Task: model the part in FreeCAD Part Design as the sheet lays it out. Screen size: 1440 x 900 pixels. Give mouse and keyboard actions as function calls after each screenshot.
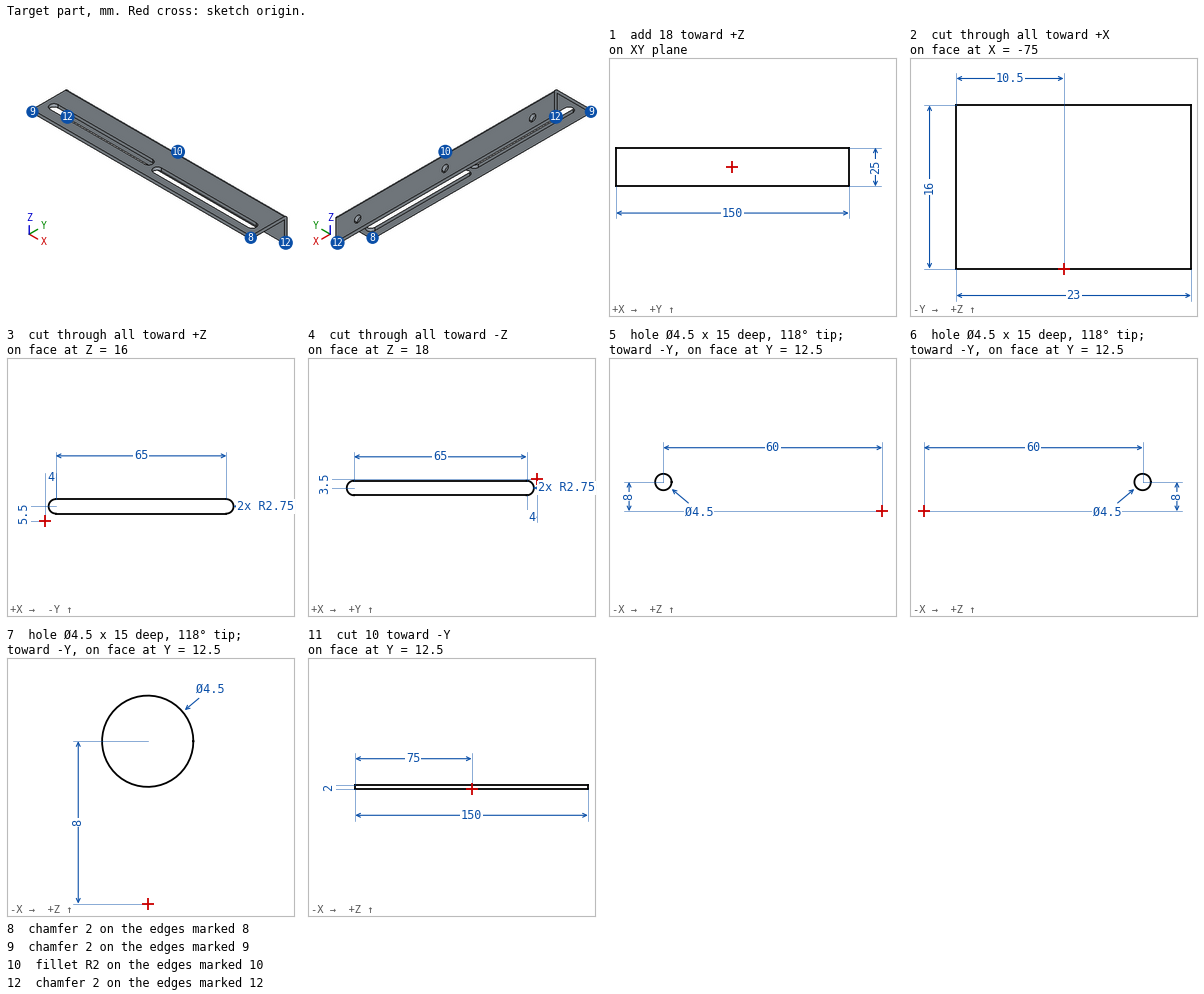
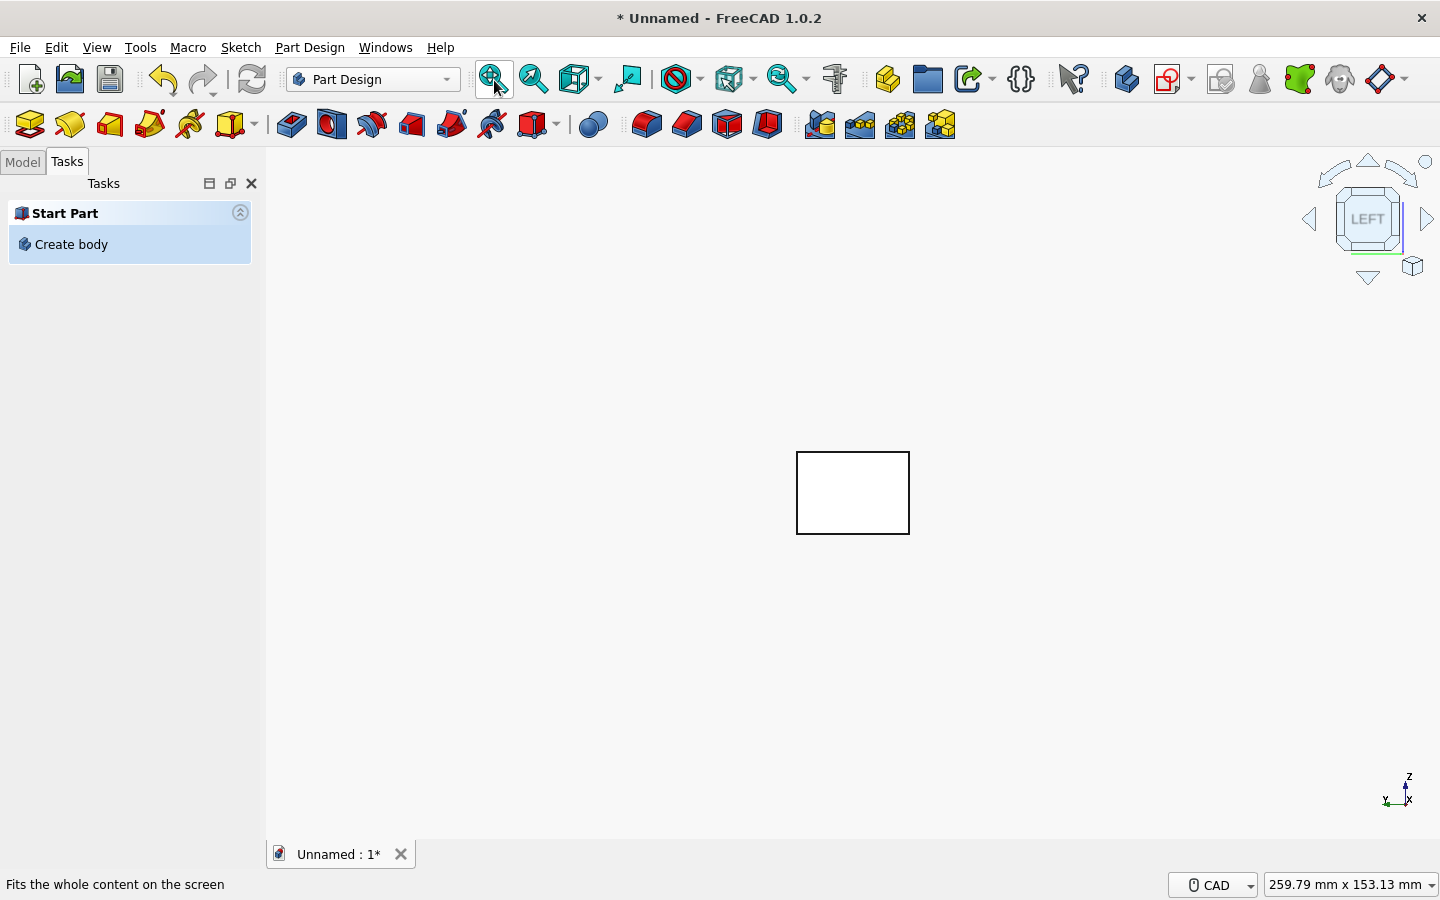
click(853, 492)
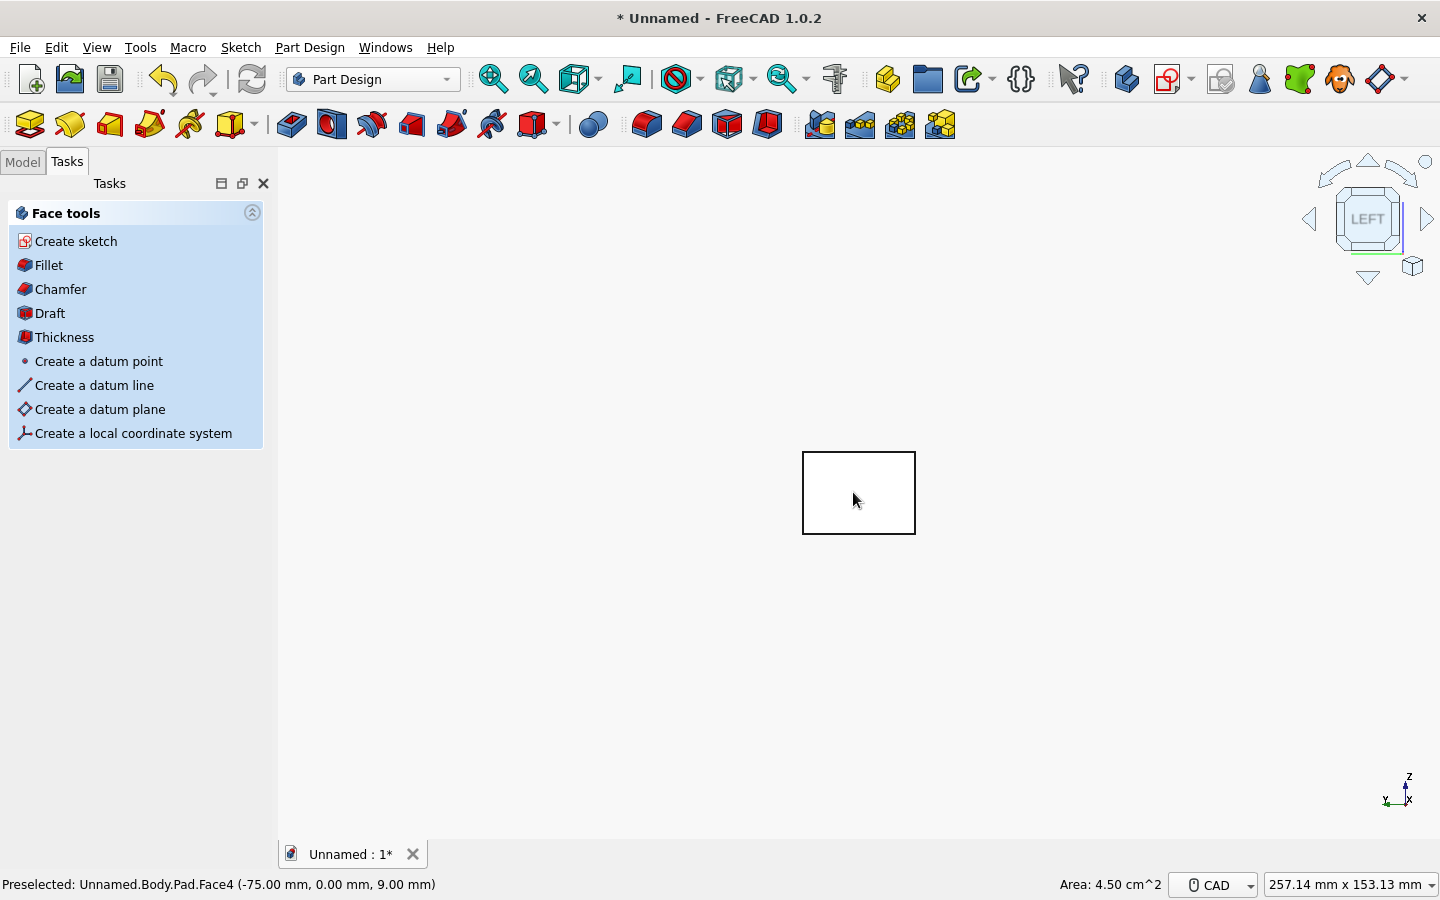
click(1168, 80)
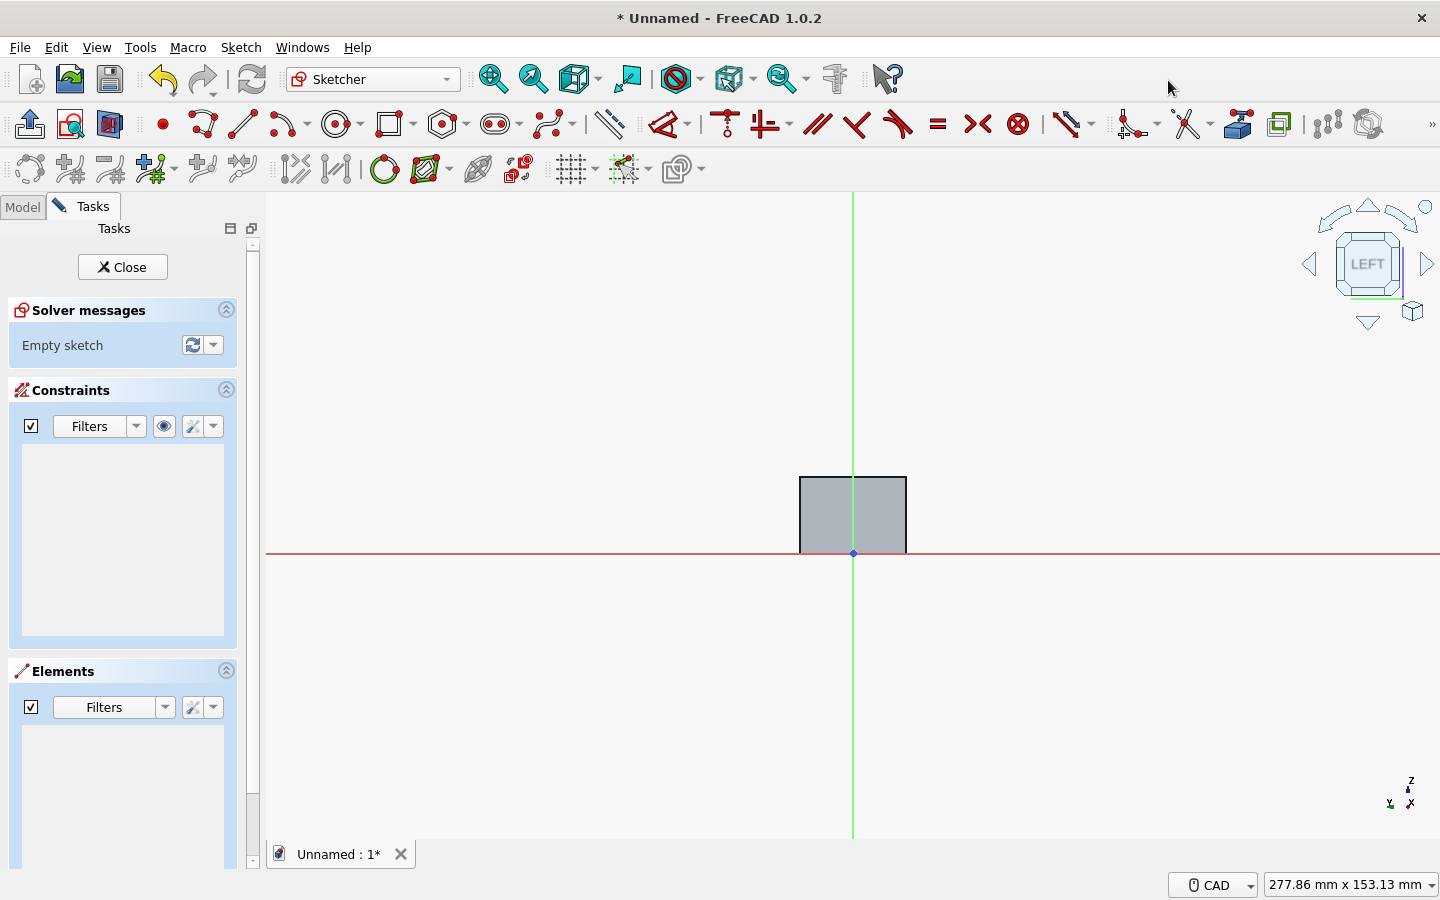
scroll(872, 521, up, 9)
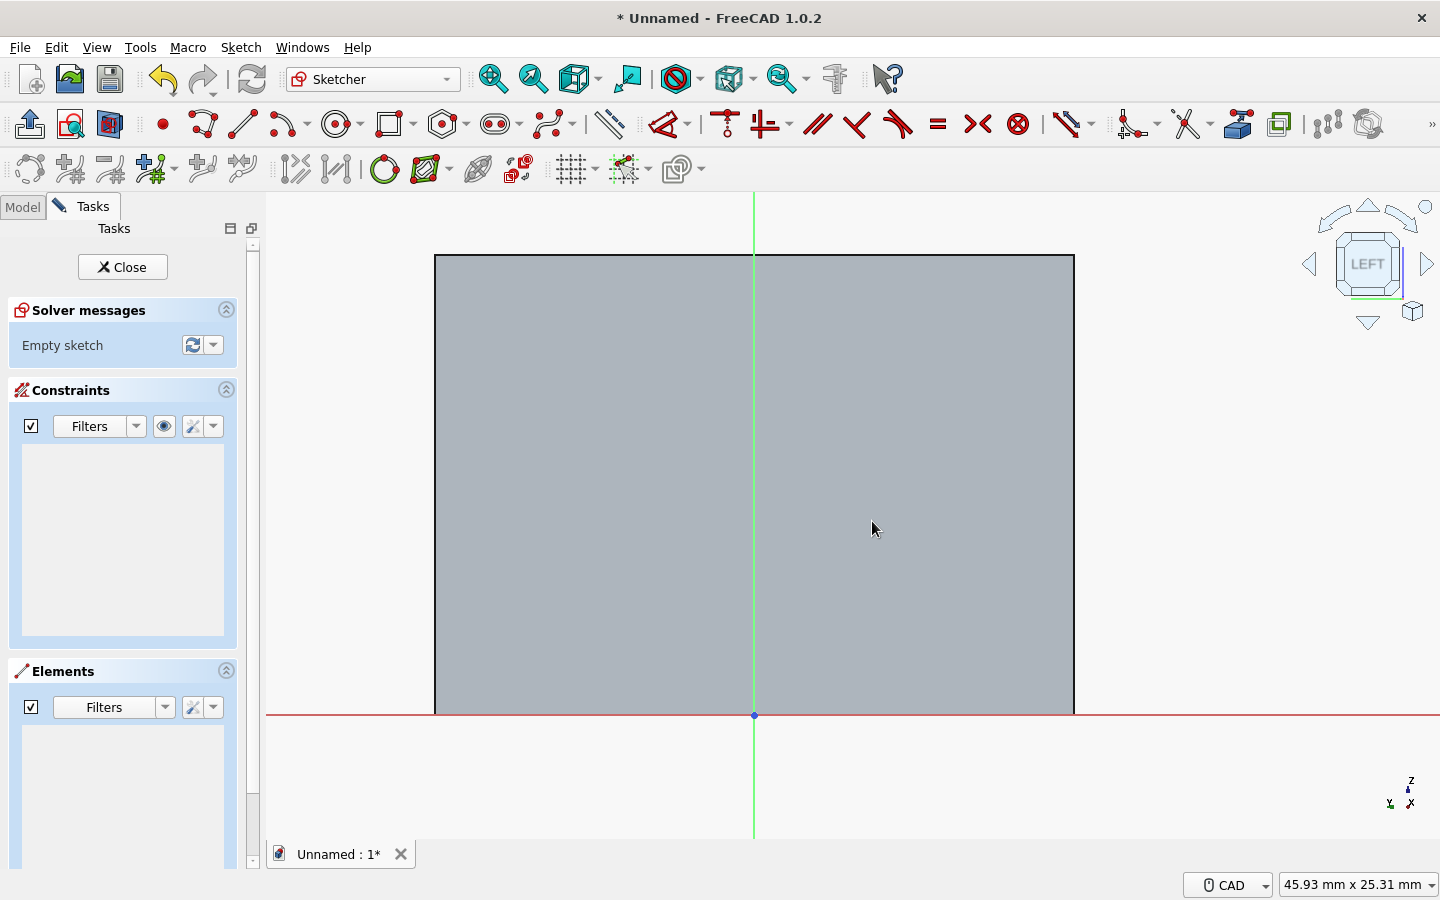
click(390, 124)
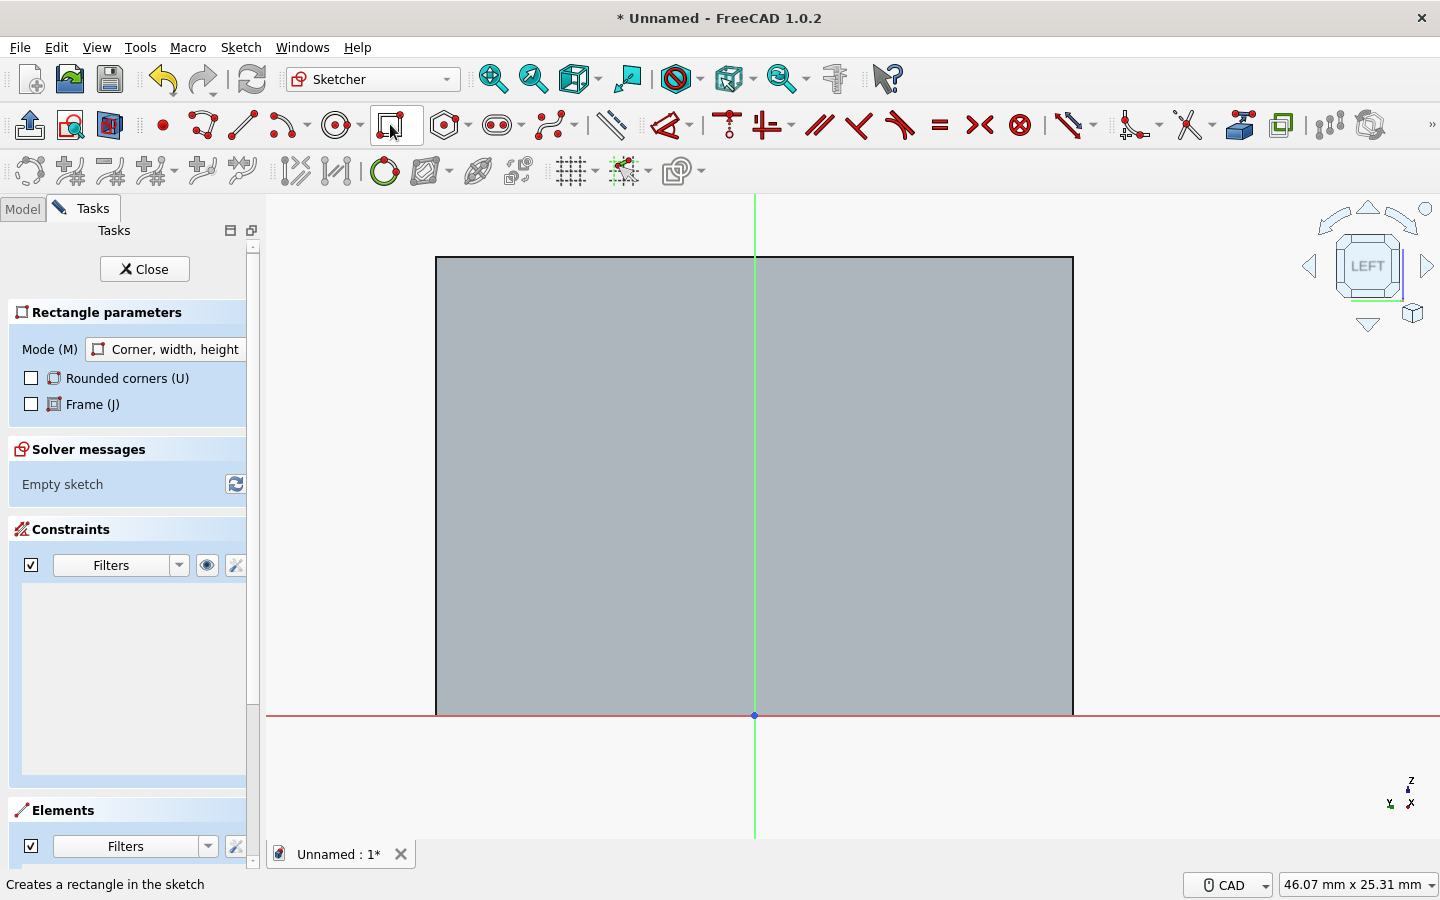
click(487, 308)
click(1073, 716)
key(Escape)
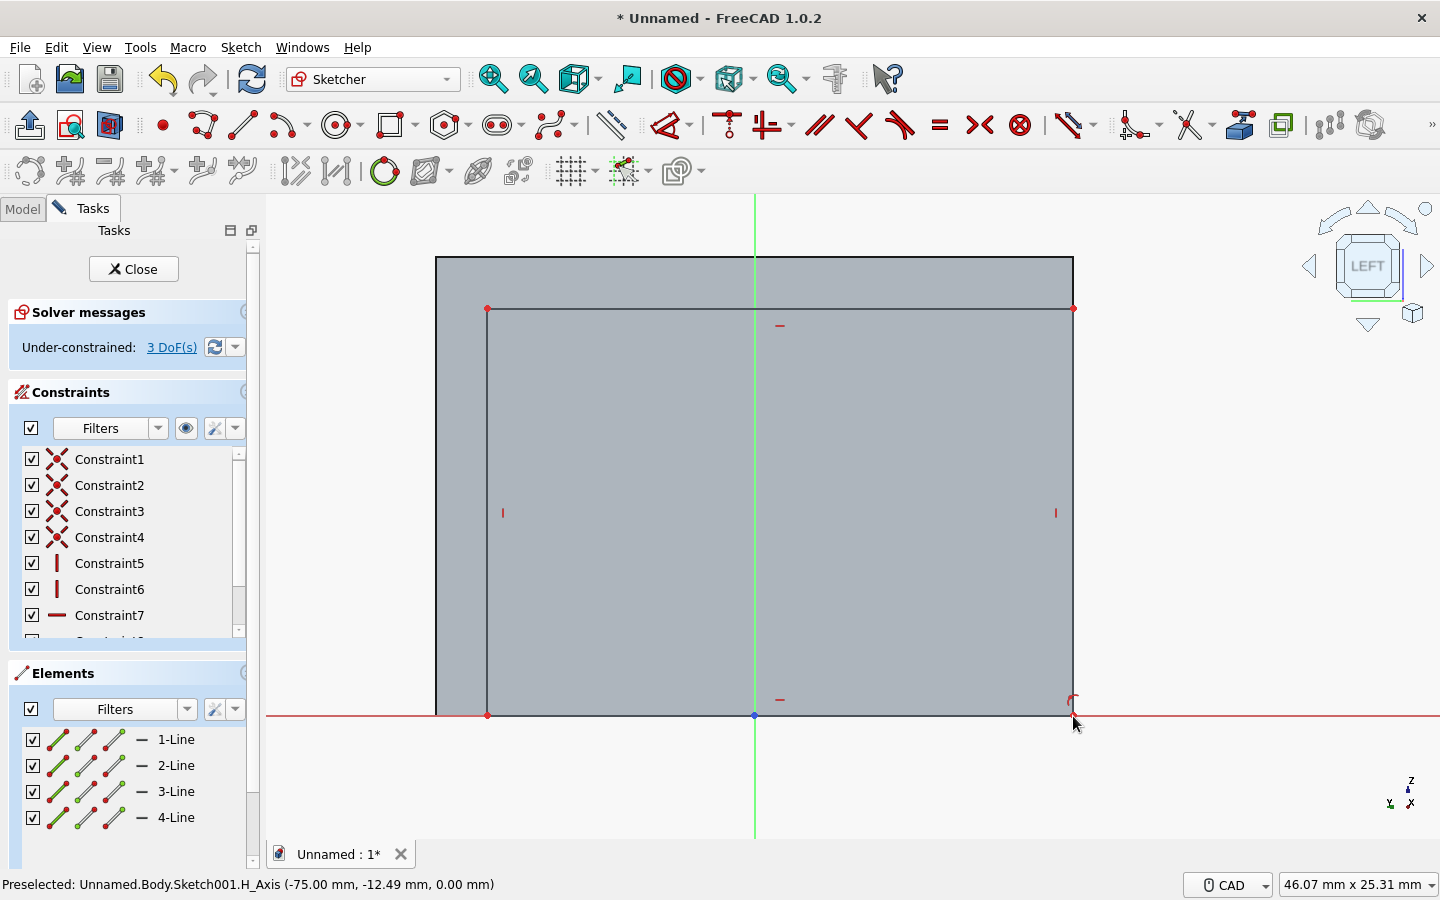
click(487, 431)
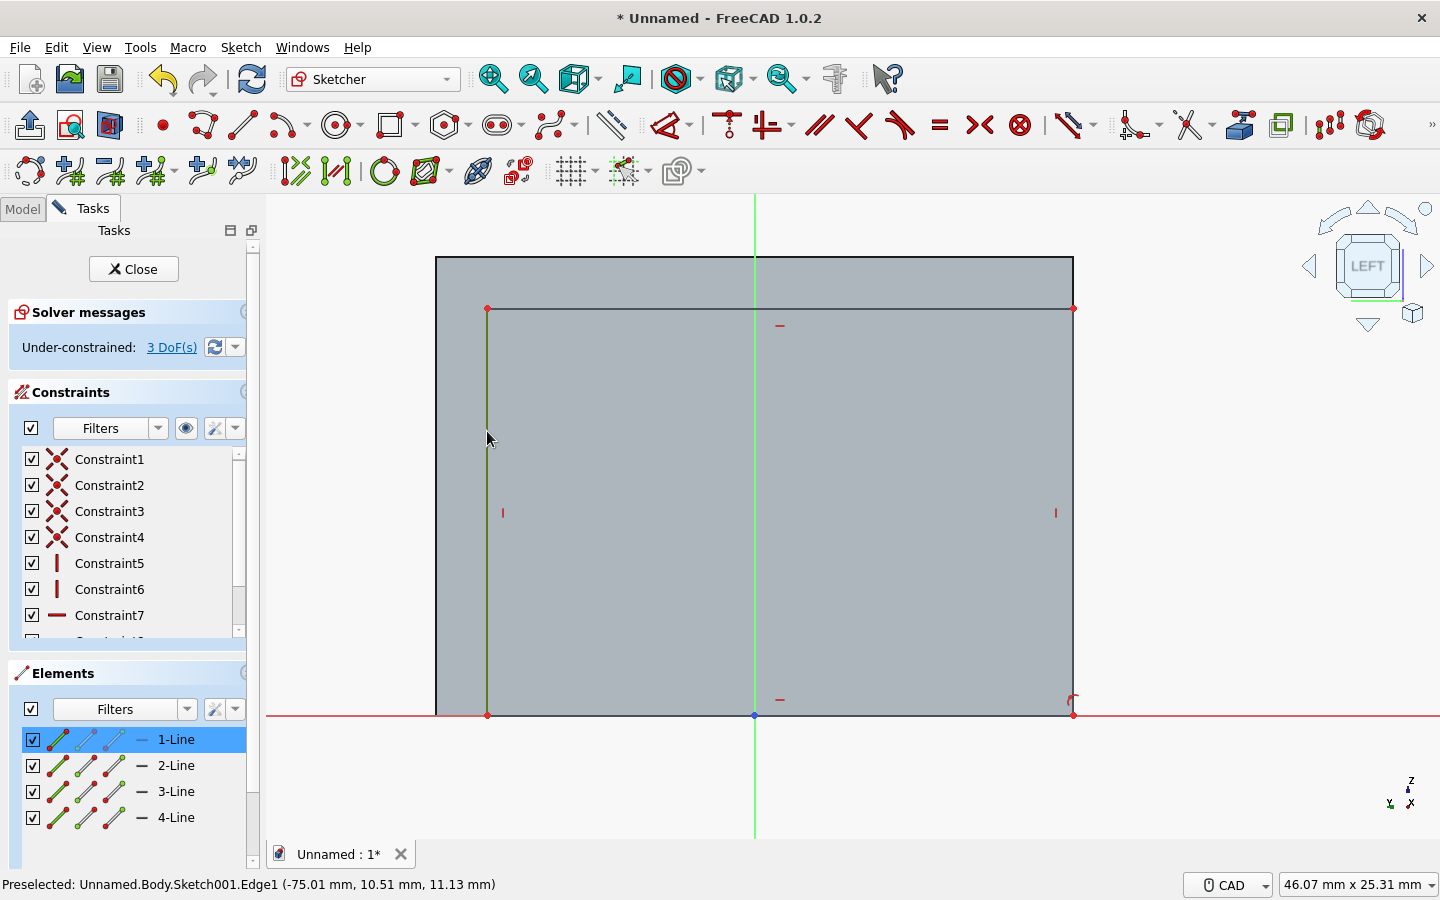
click(692, 126)